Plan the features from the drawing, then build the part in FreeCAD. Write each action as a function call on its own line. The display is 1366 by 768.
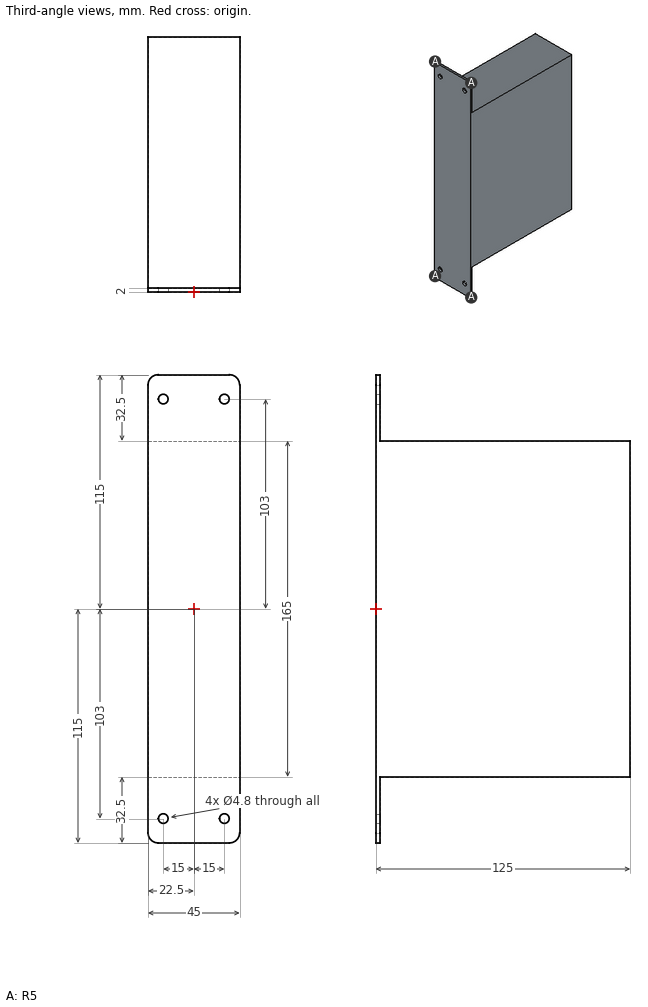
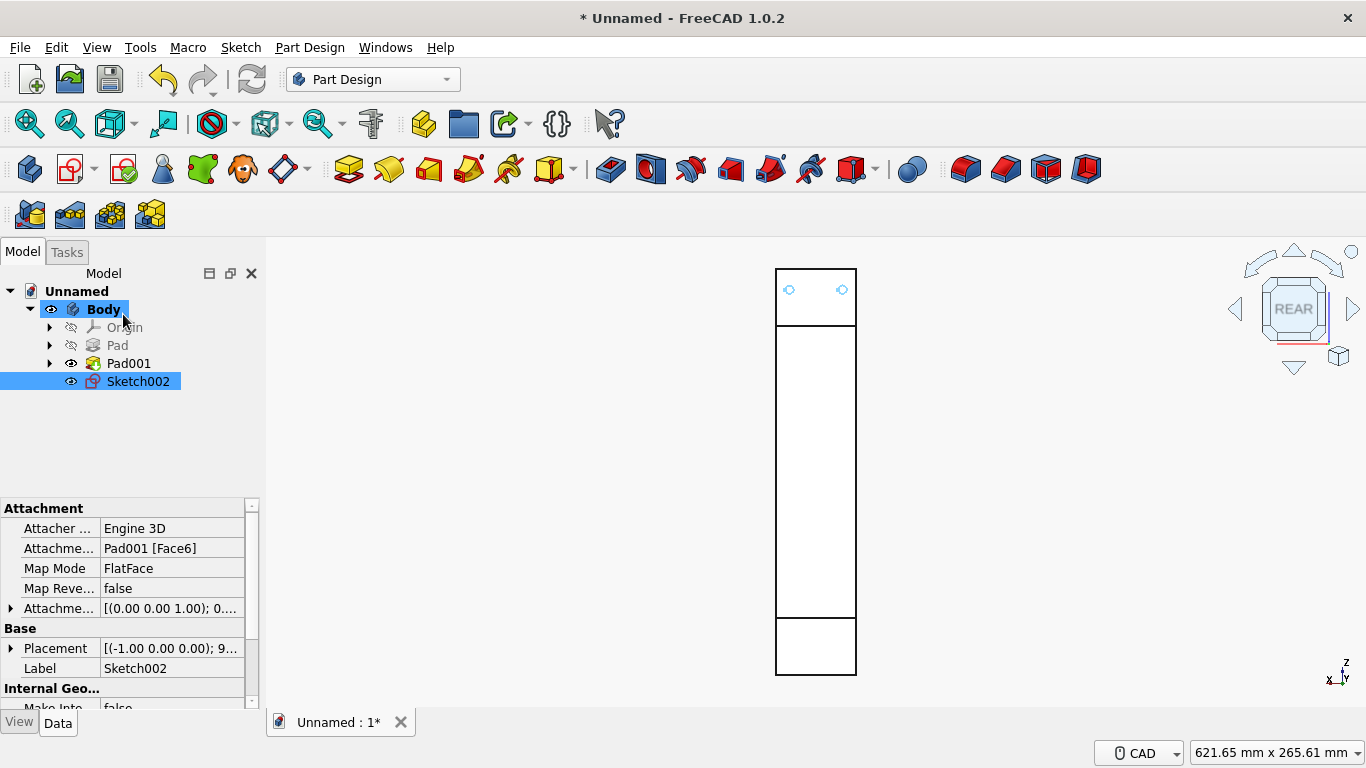
click(652, 170)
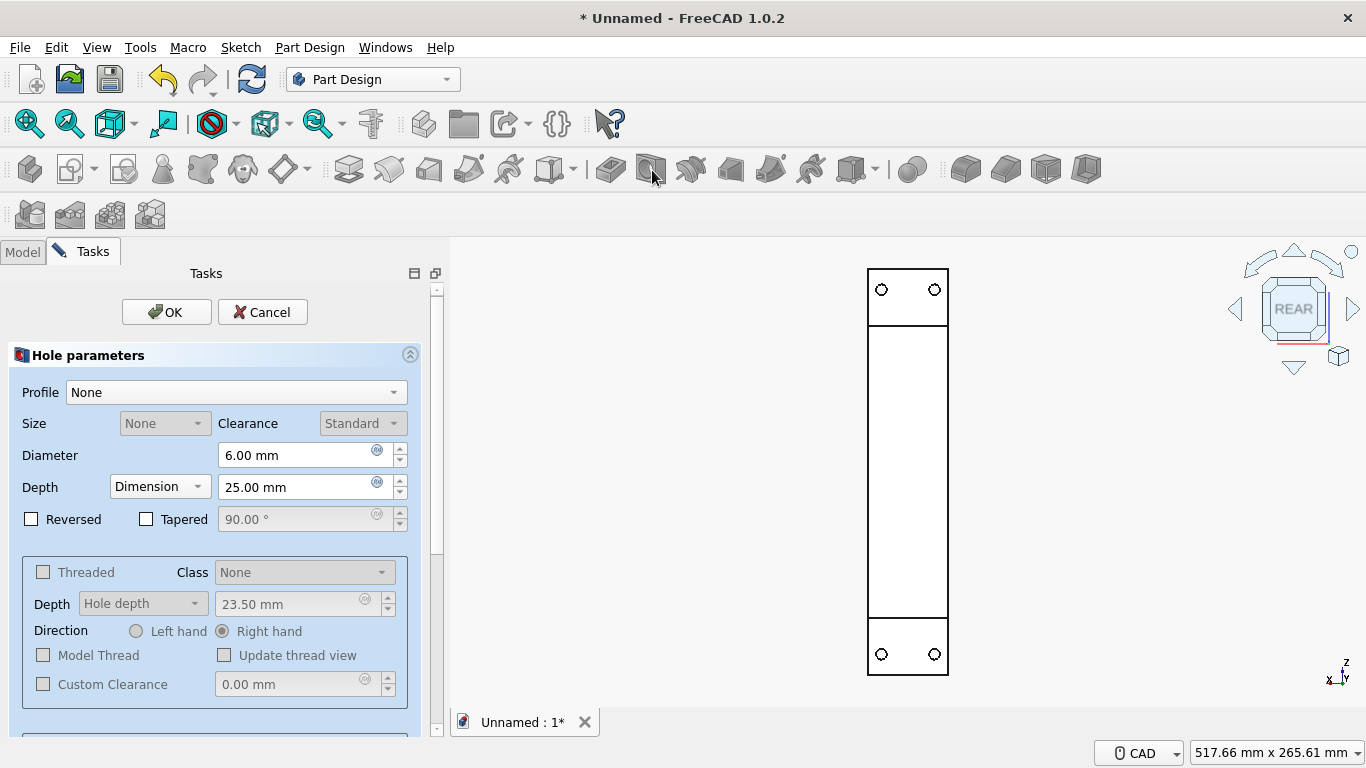
triple_click(305, 455)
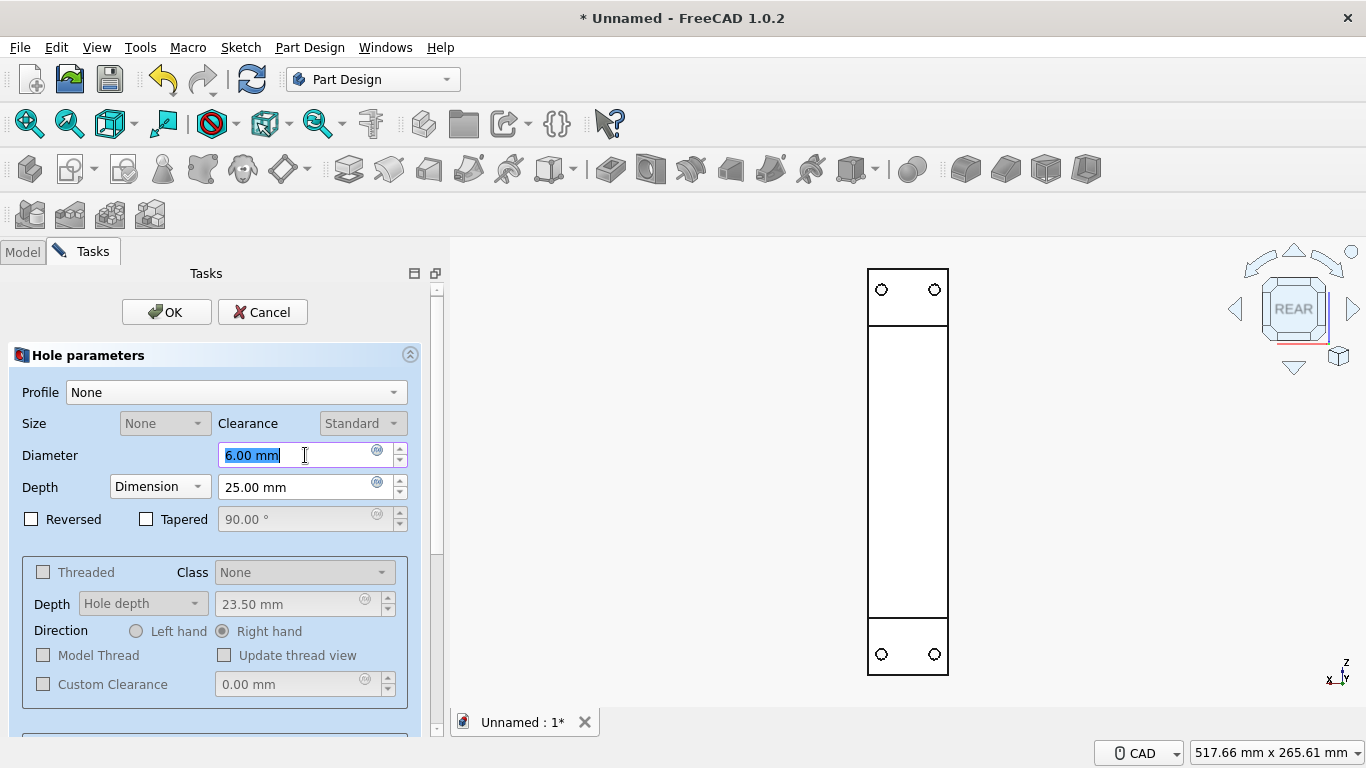
text(4.8)
key(Tab)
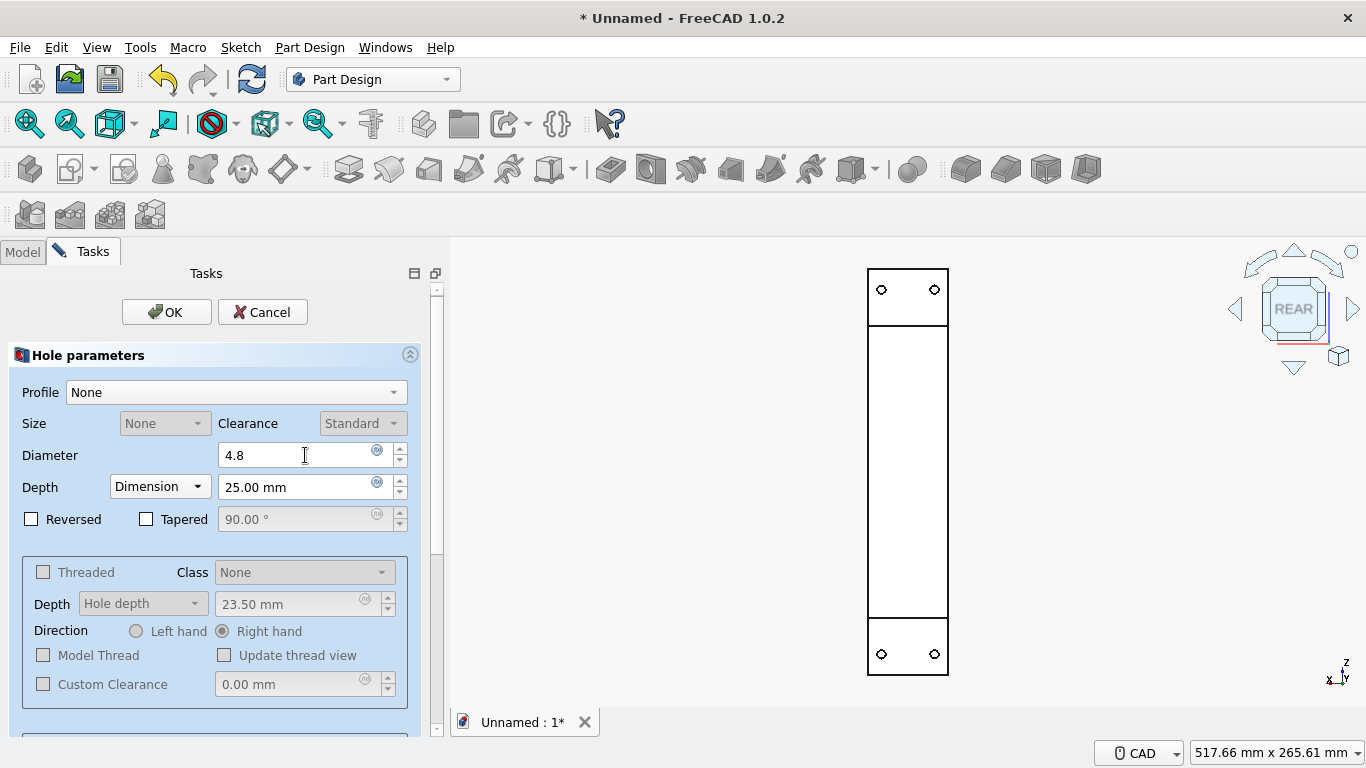
click(161, 486)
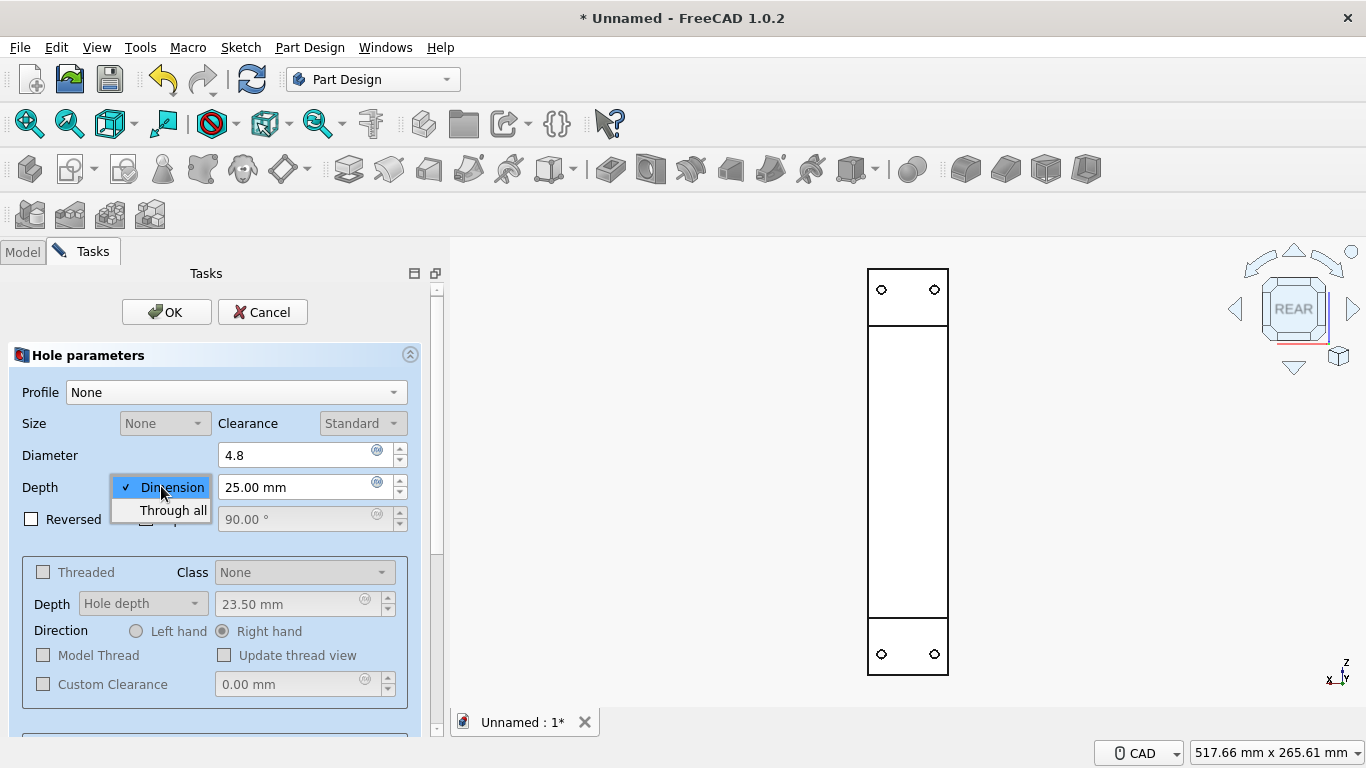
click(160, 510)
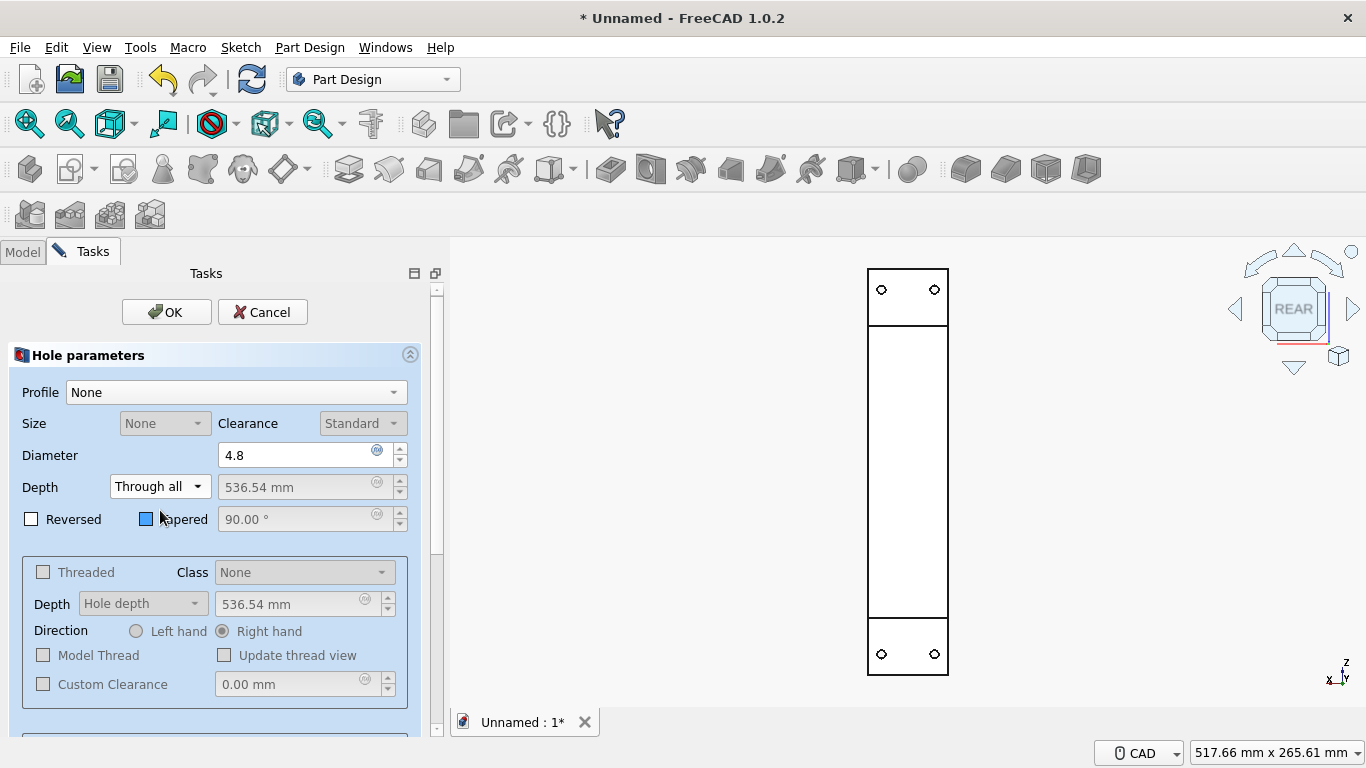
click(167, 312)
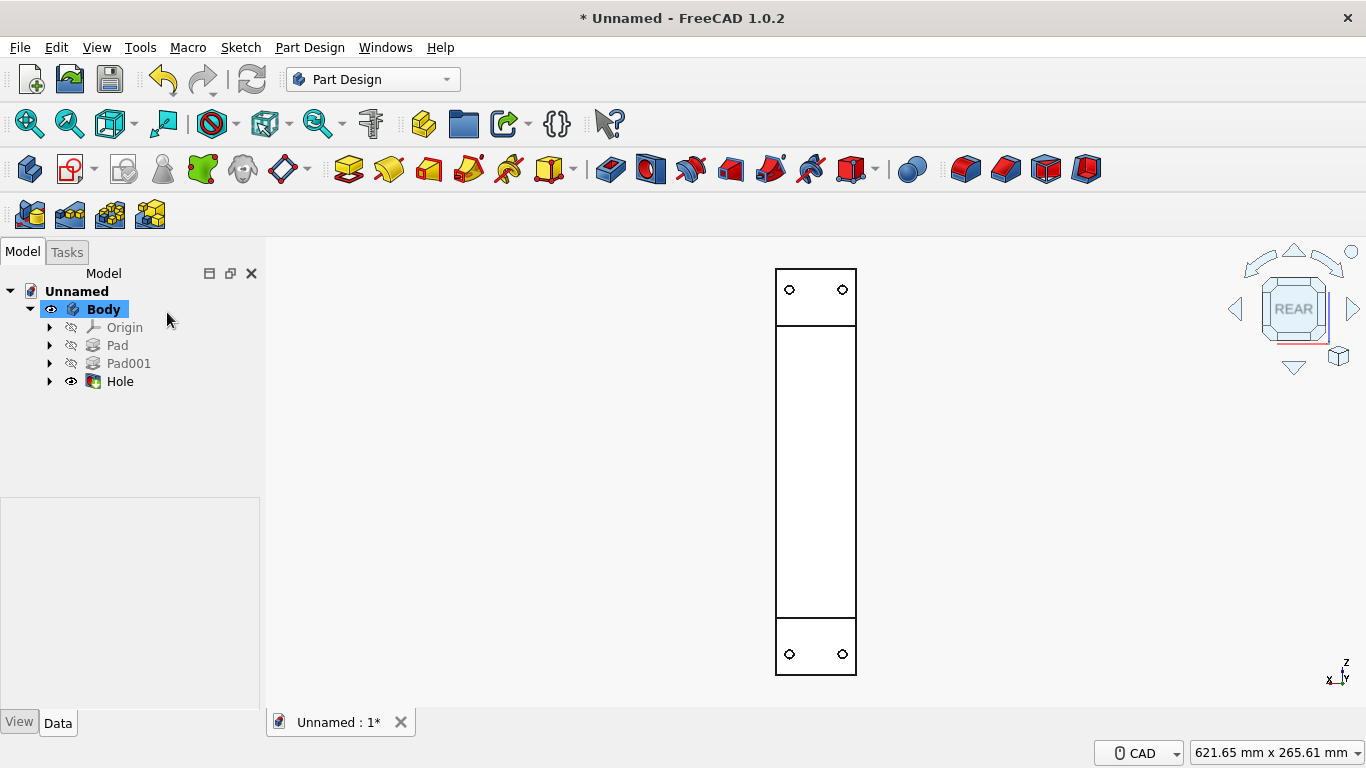
scroll(856, 674, up, 13)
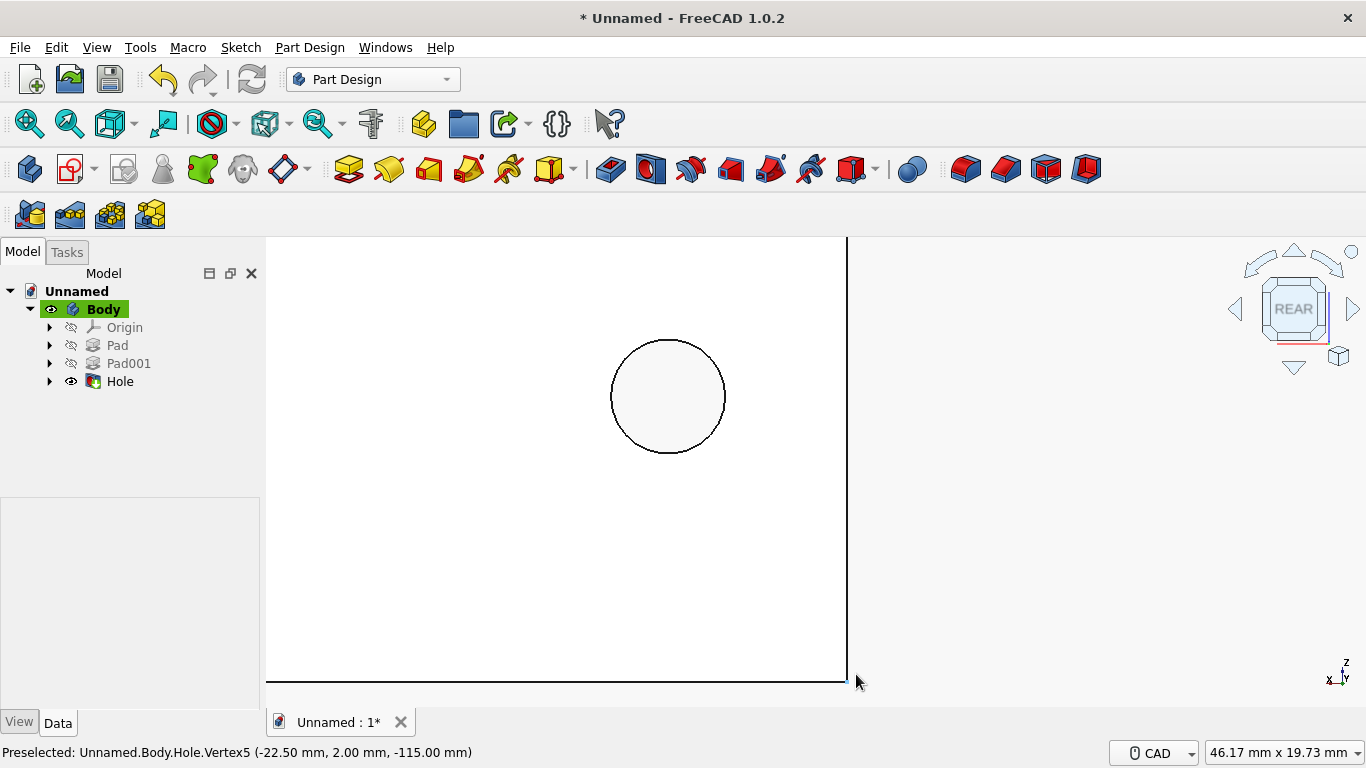
key(v)
key(f)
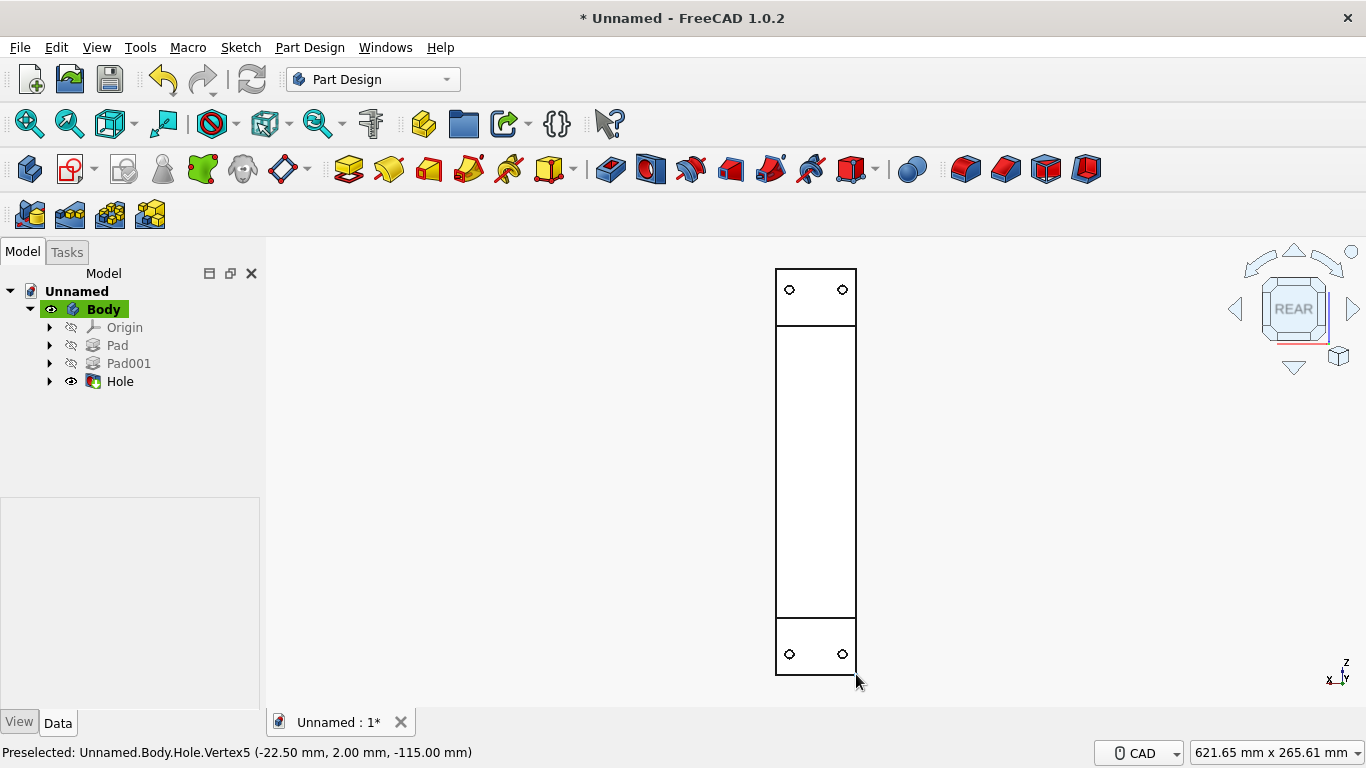
key(0)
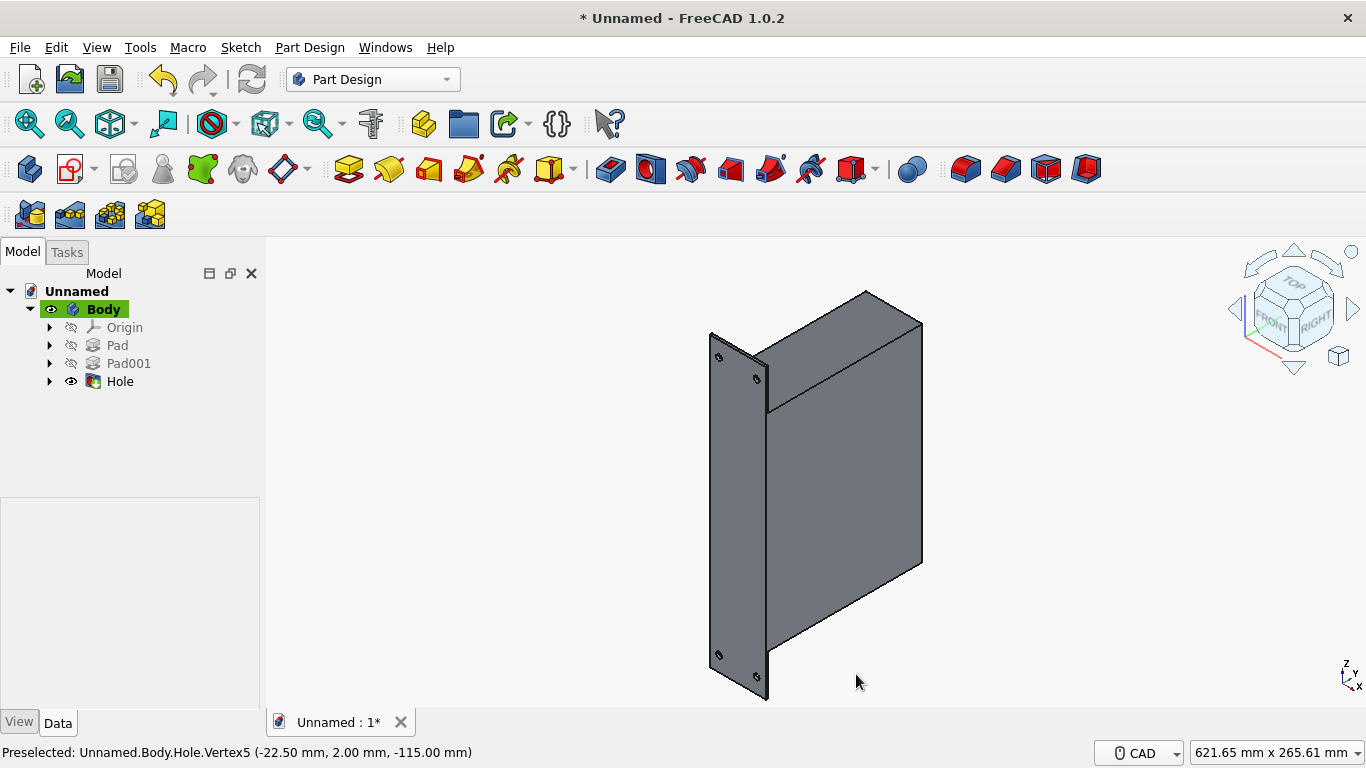
scroll(711, 665, up, 13)